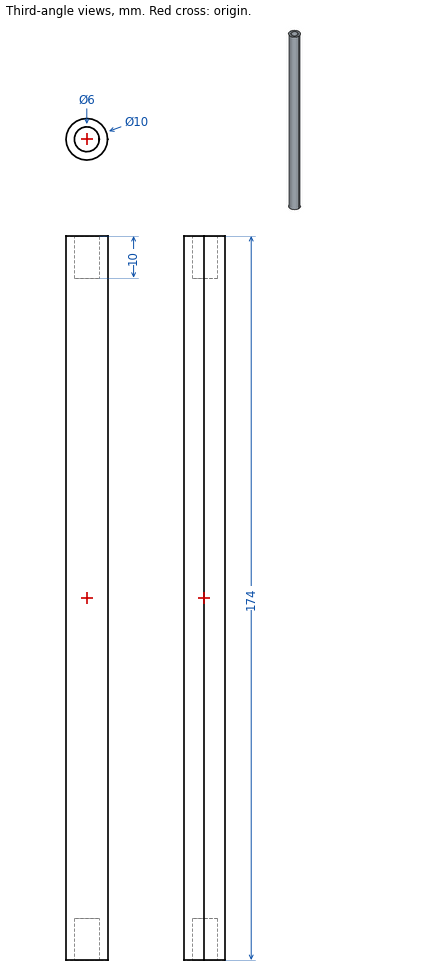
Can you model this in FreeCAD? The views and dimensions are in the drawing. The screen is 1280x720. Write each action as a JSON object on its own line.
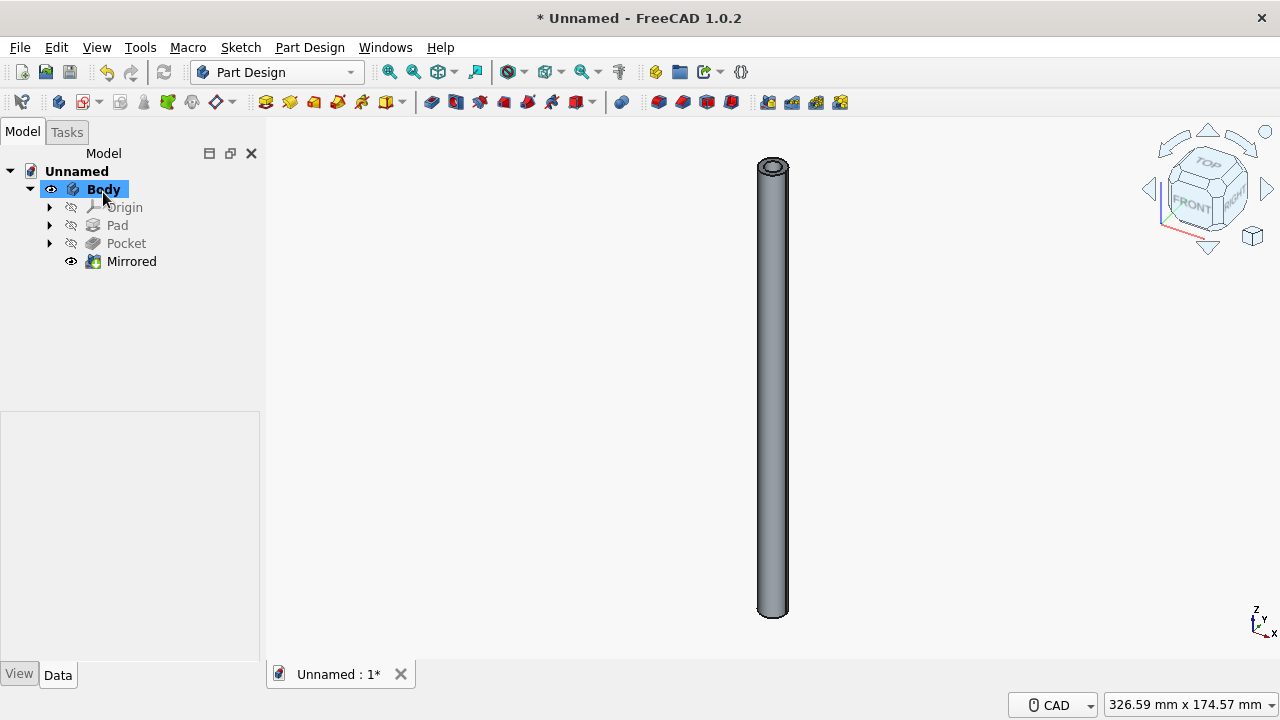
{"action": "key", "text": "0"}